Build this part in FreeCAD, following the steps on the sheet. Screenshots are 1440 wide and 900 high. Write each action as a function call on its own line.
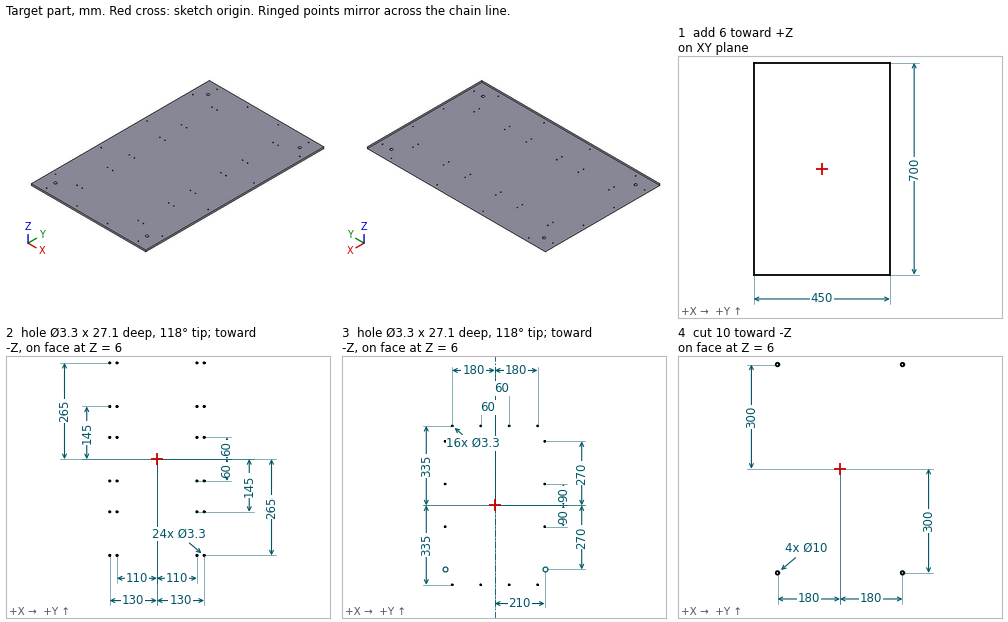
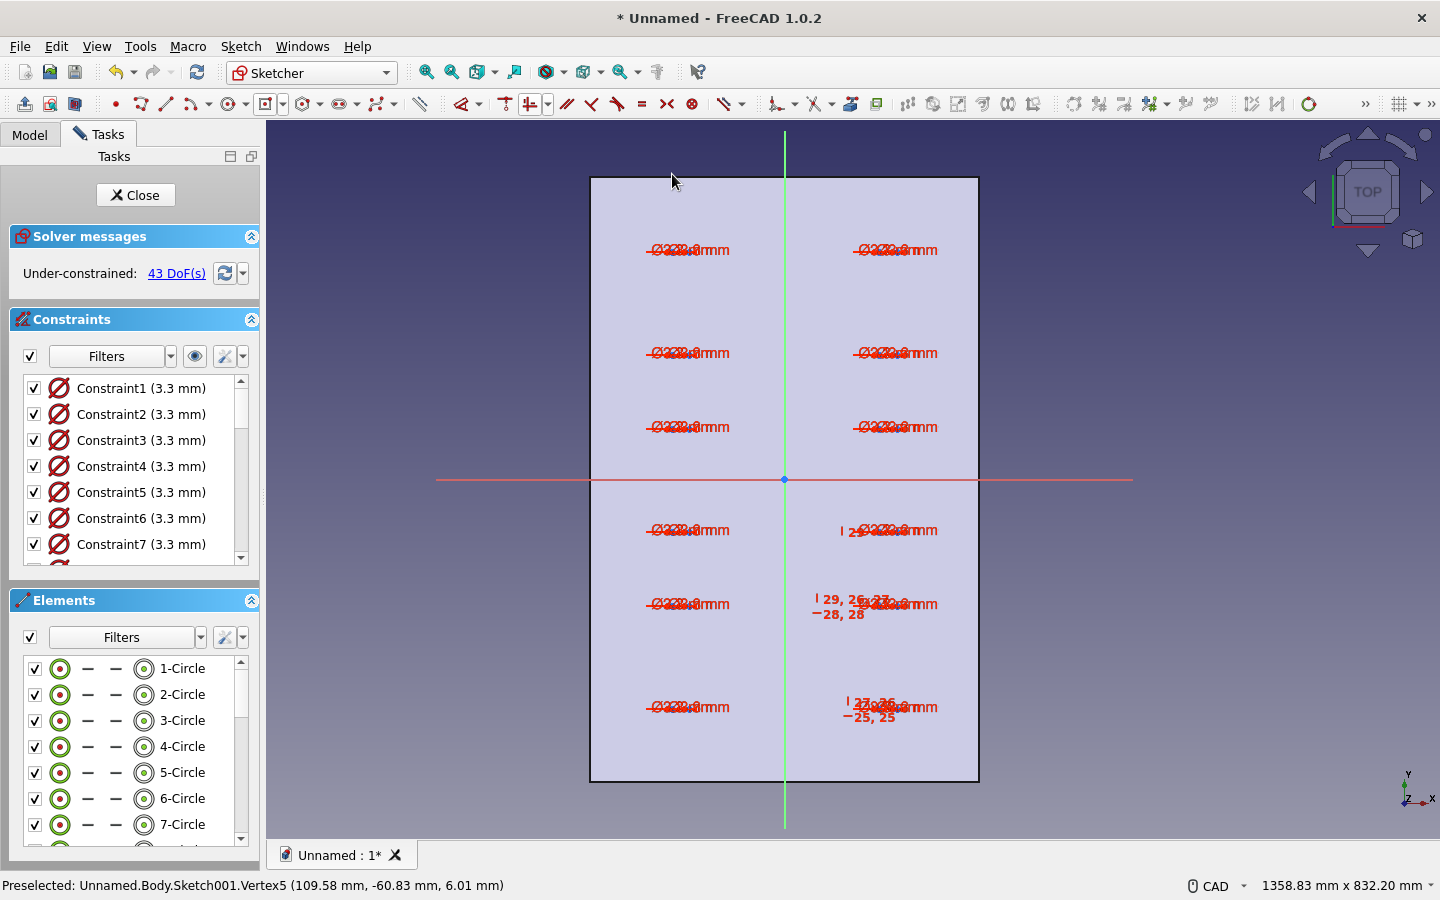
click(897, 606)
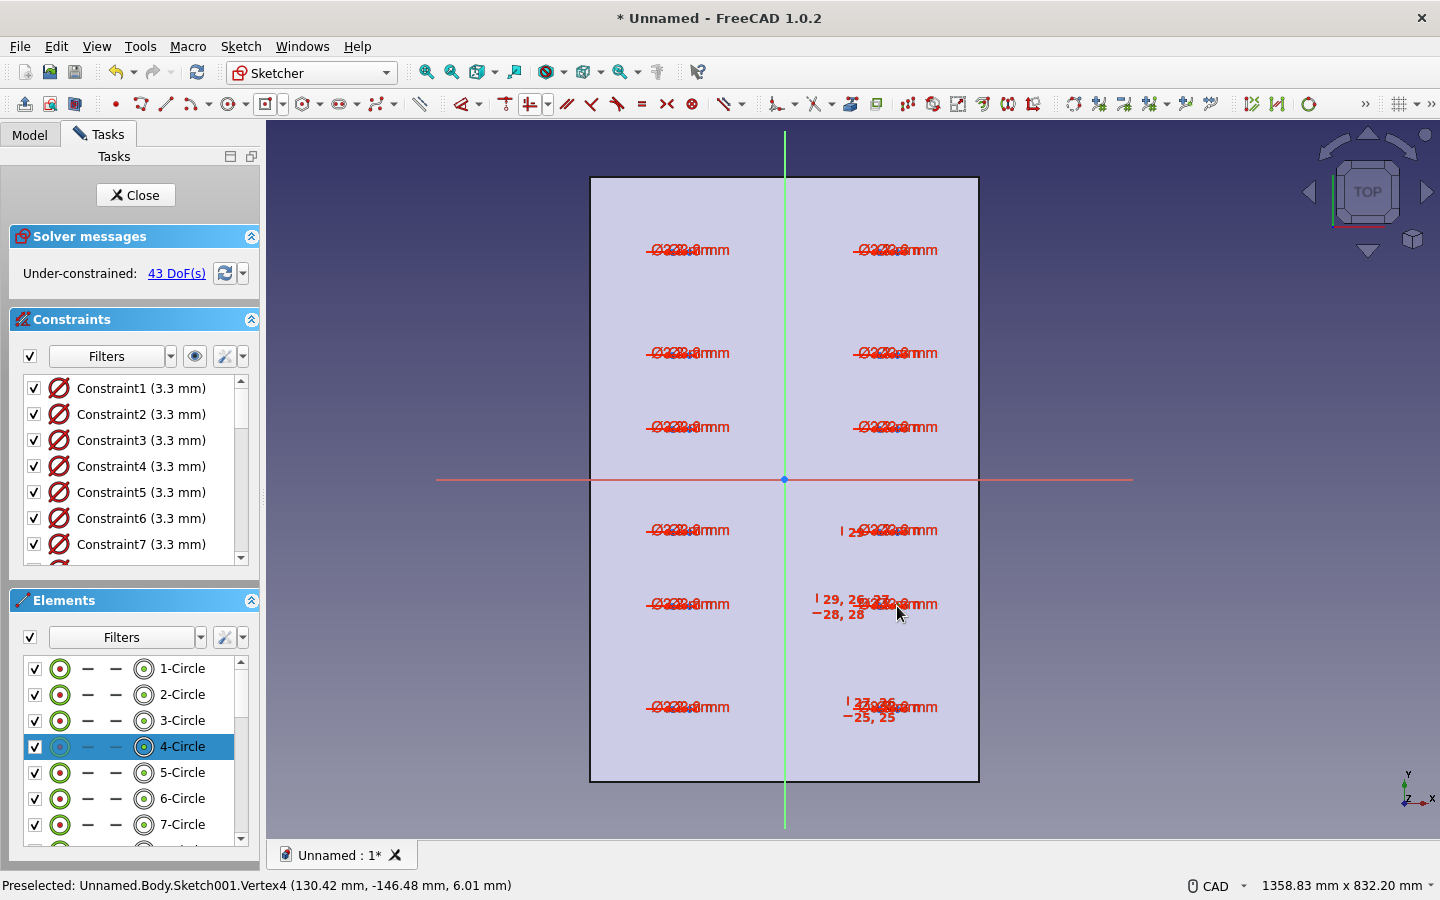
click(897, 532)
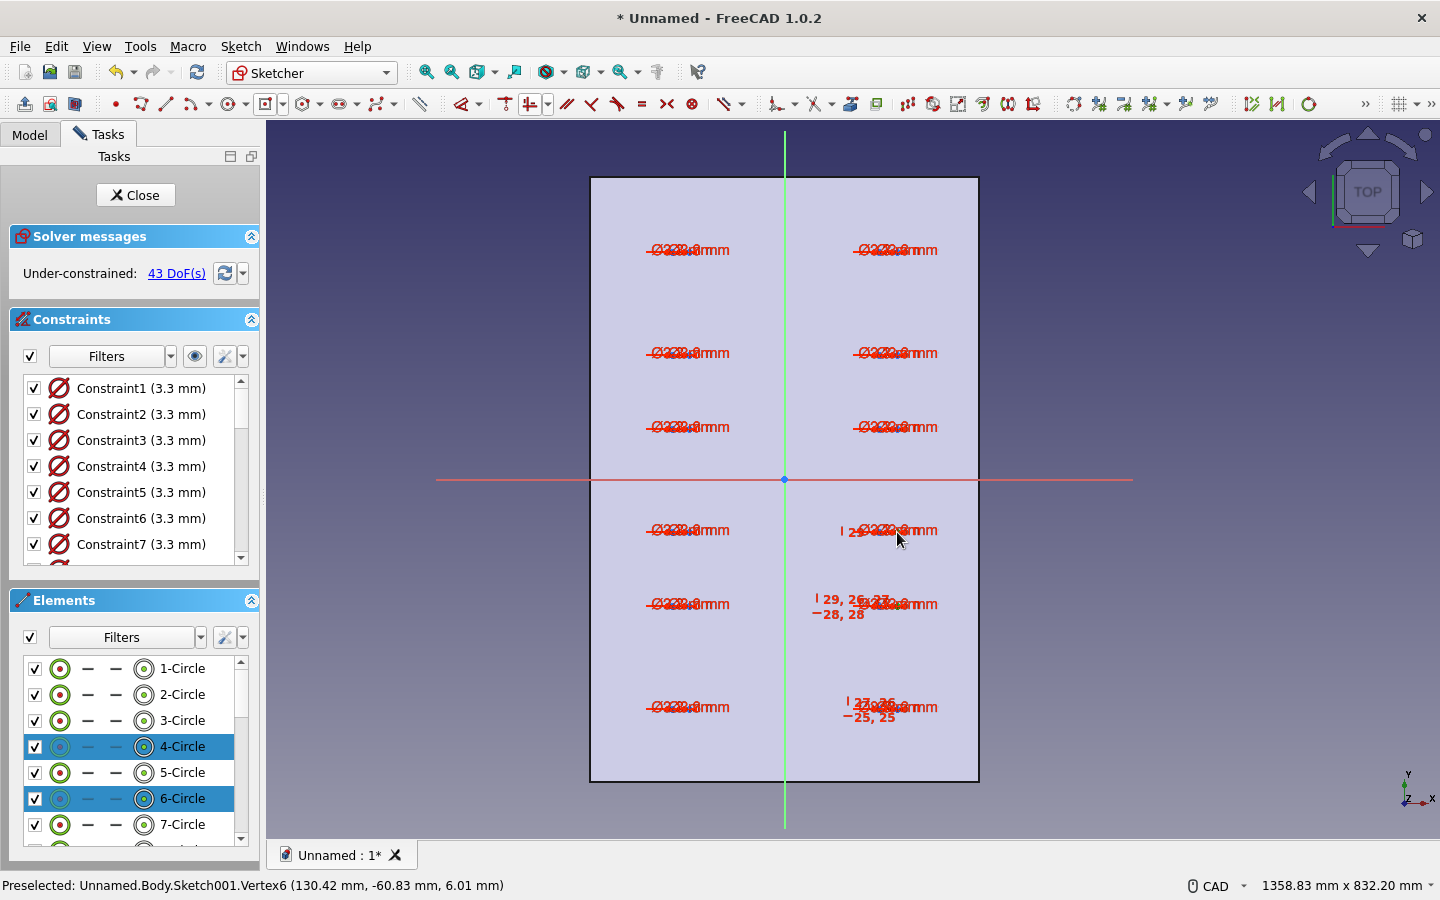
click(548, 104)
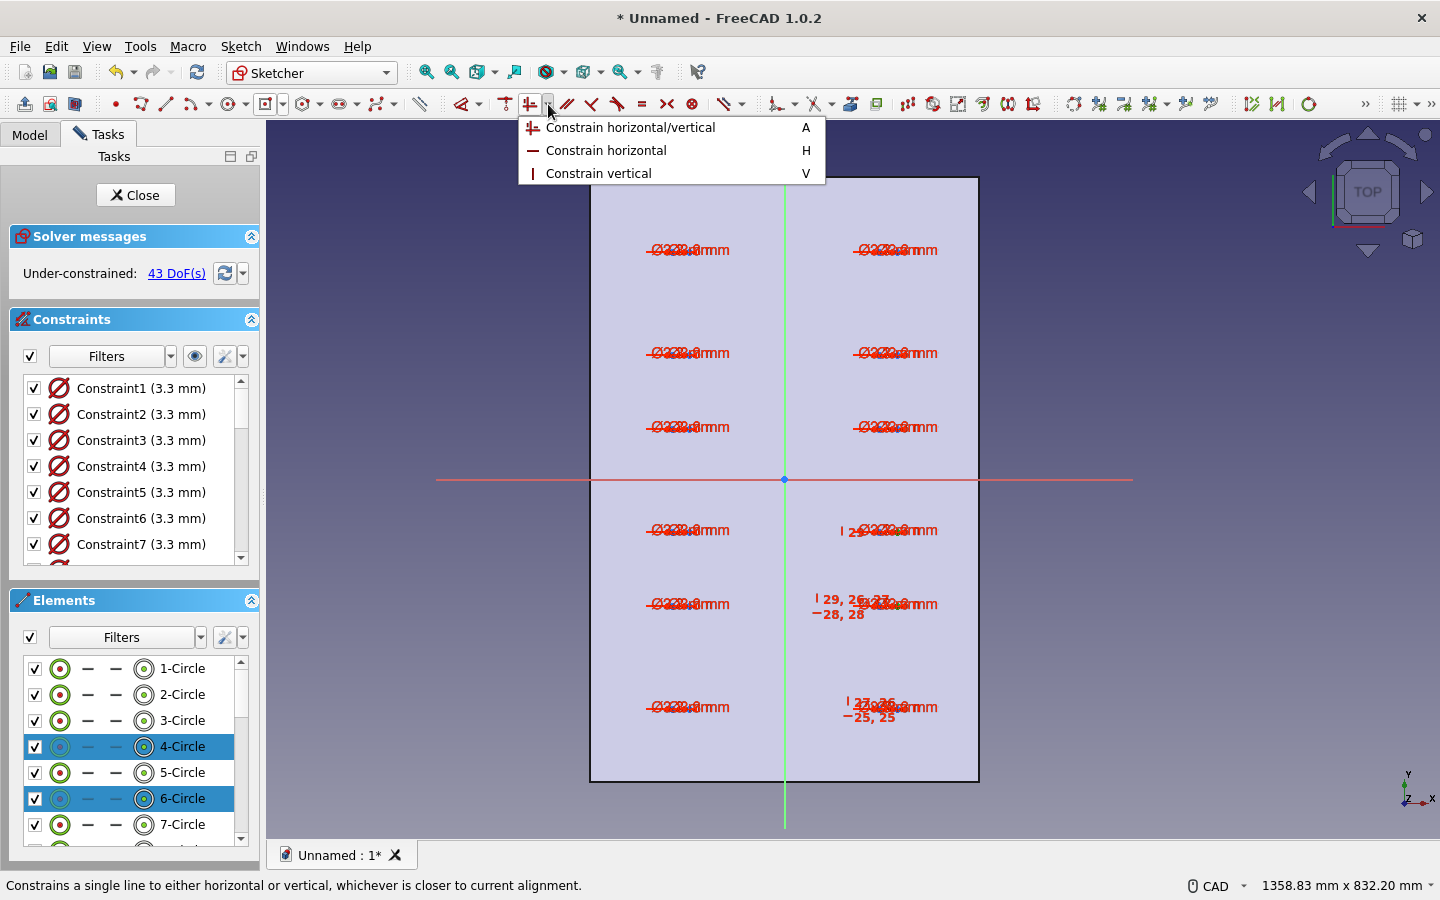
click(672, 174)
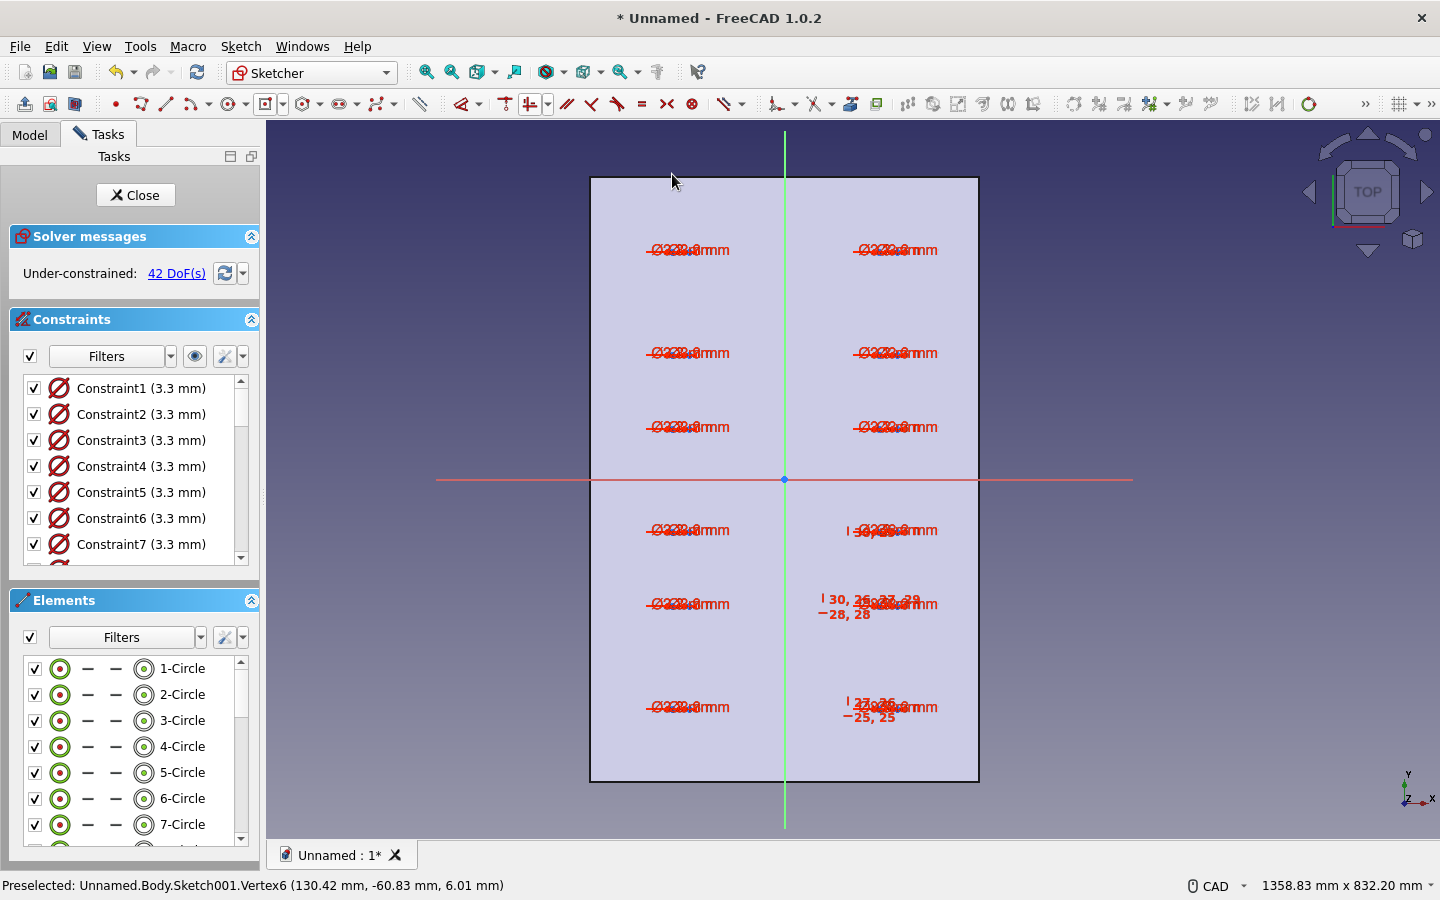
scroll(879, 532, up, 4)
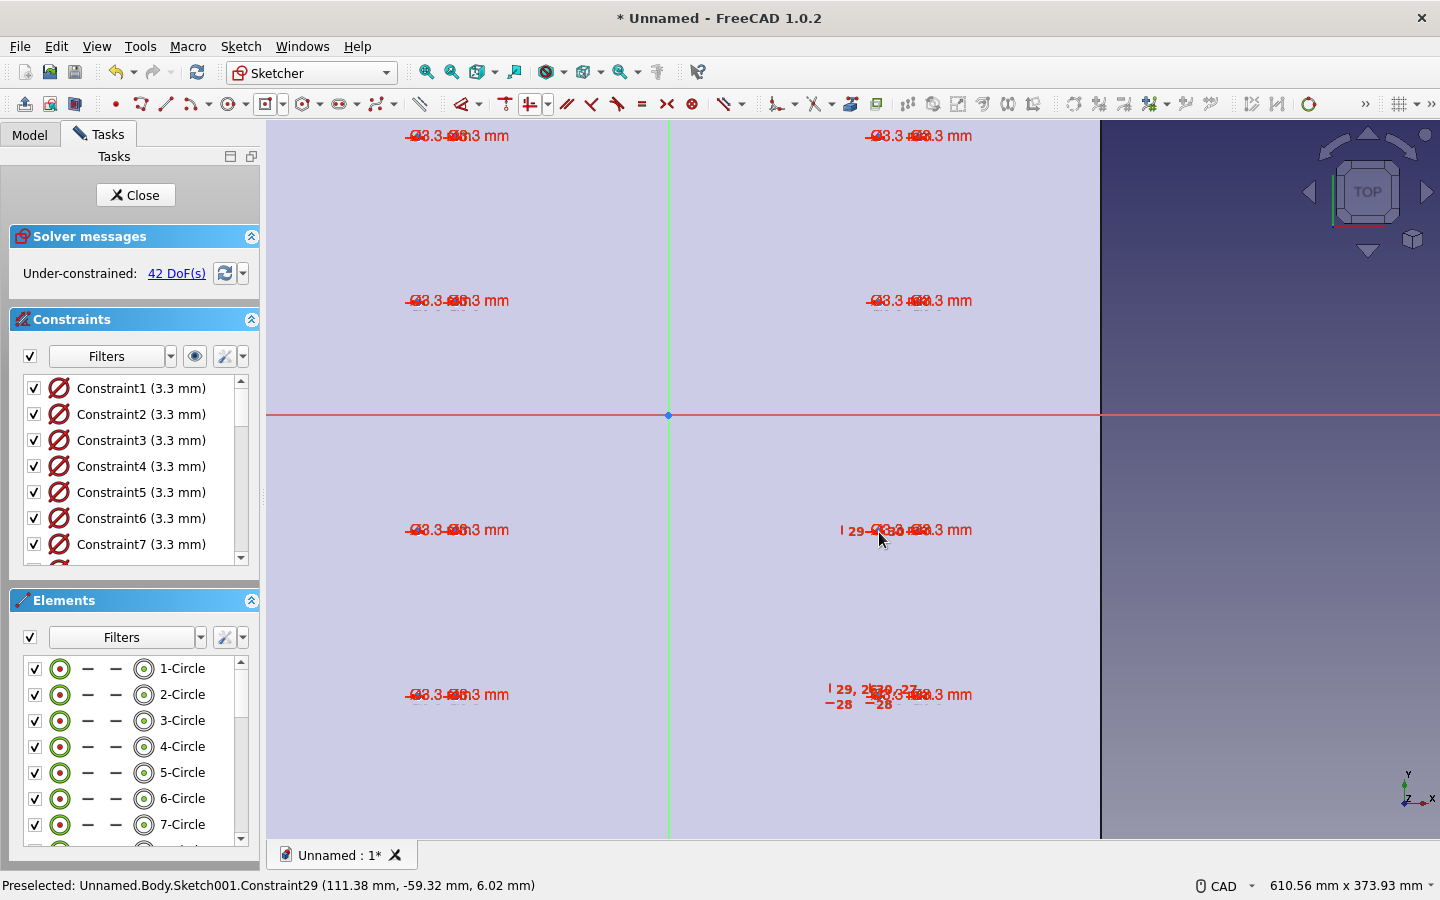
scroll(879, 532, up, 4)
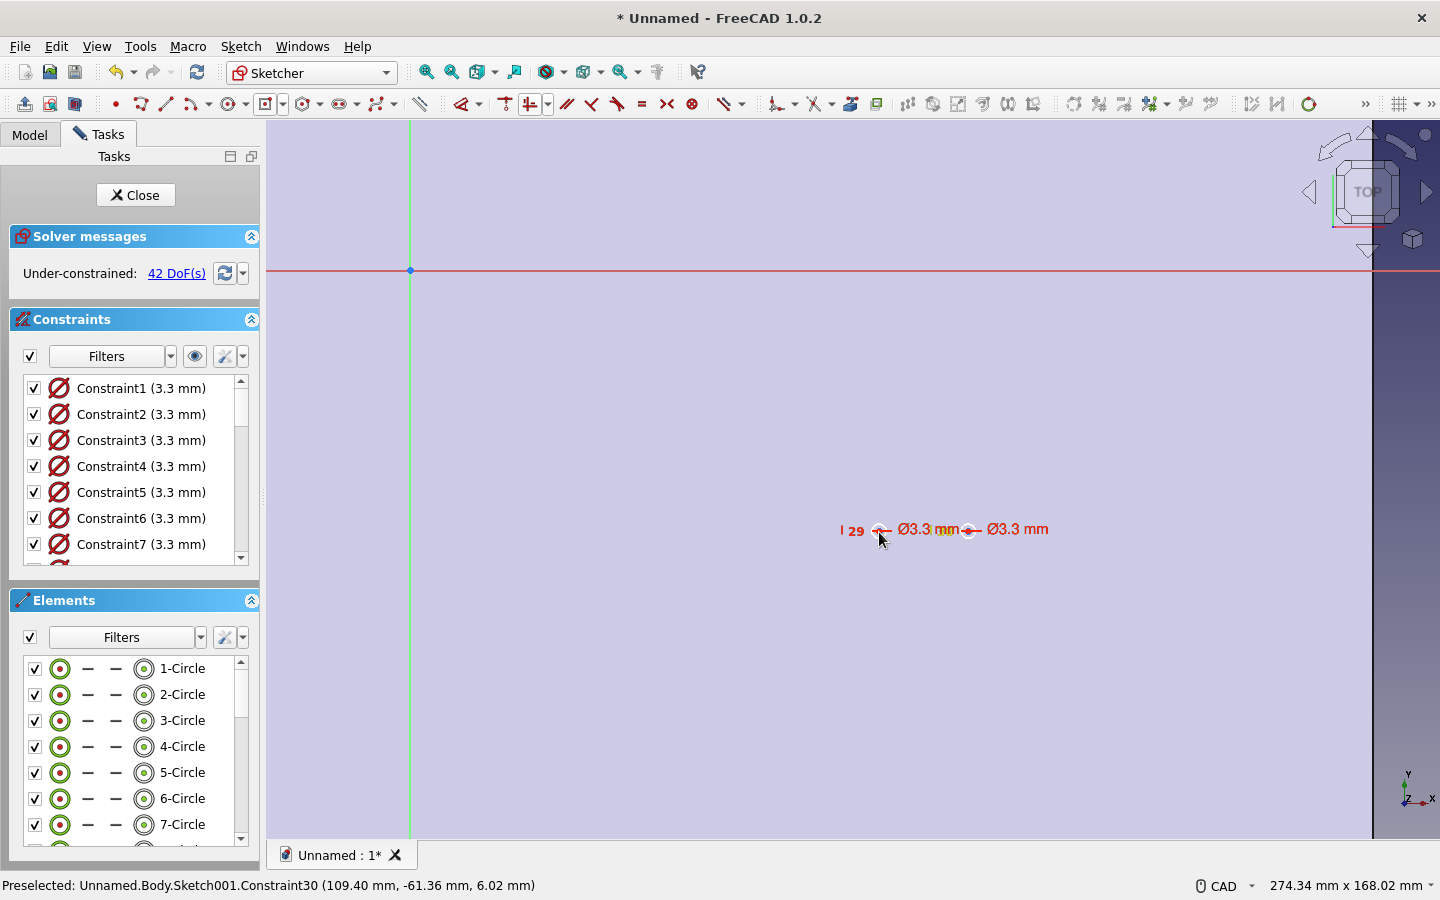
click(879, 531)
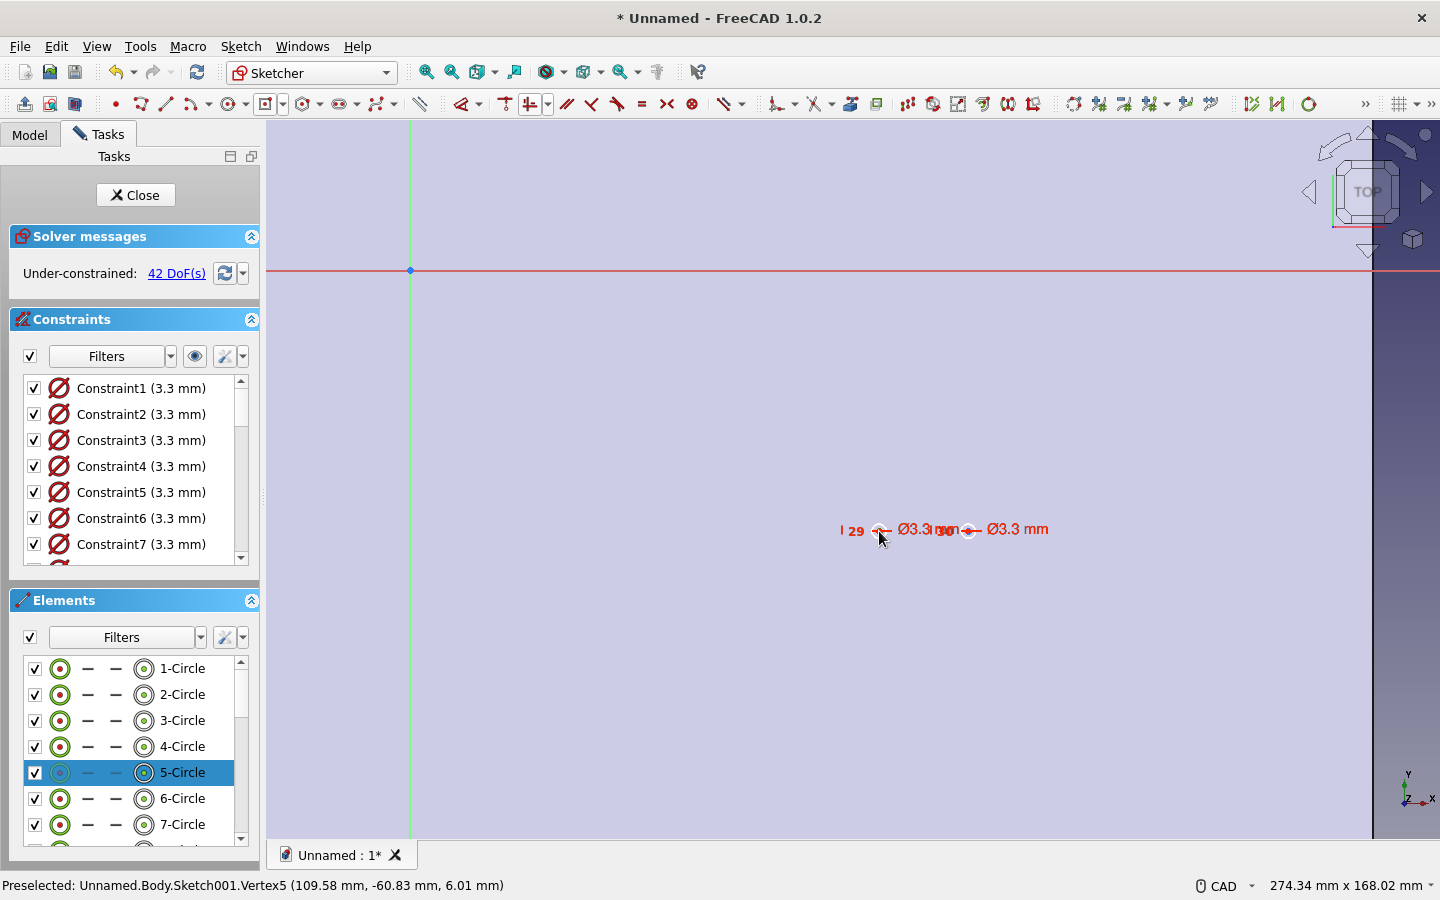
scroll(879, 532, down, 8)